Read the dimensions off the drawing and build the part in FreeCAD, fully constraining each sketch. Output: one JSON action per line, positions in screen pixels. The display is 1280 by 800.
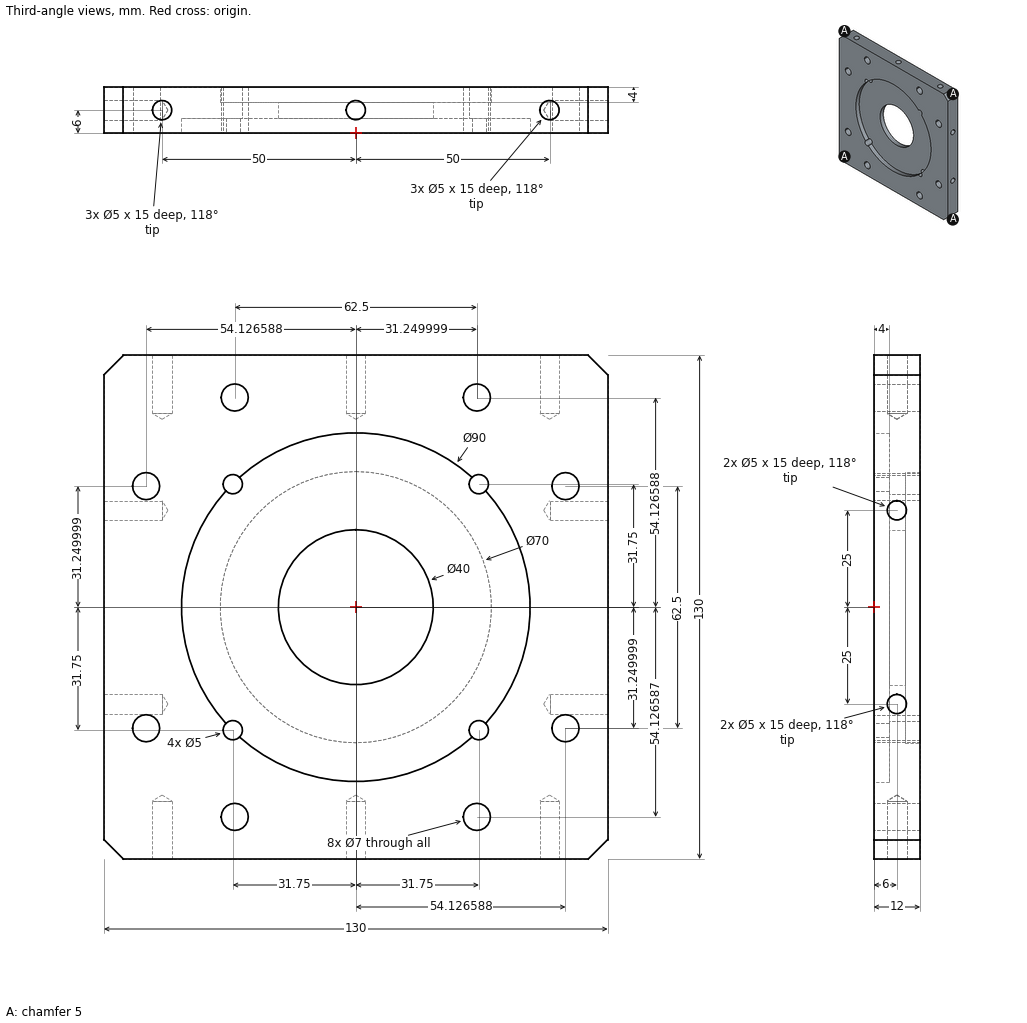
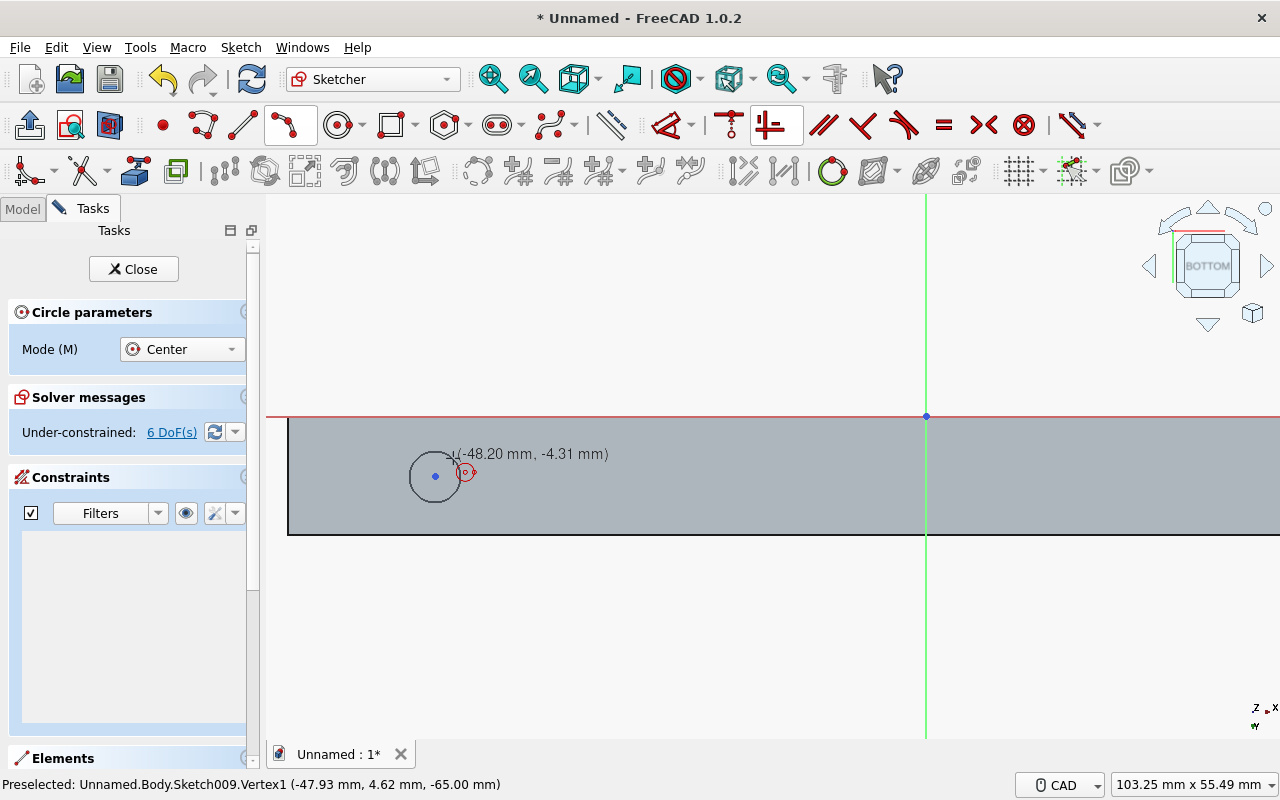
{"action": "left_click", "coordinate": [926, 476]}
{"action": "left_click", "coordinate": [944, 458]}
{"action": "key", "text": "Escape"}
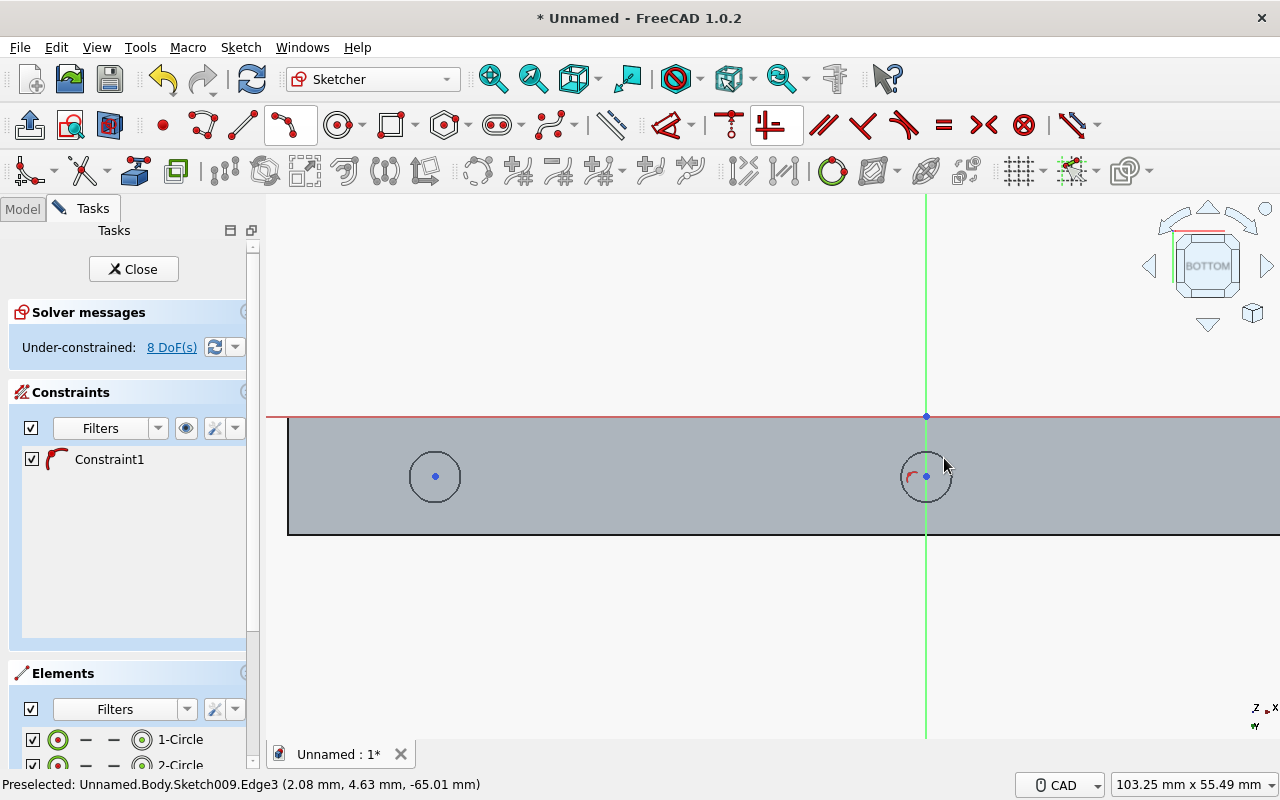
{"action": "scroll", "coordinate": [435, 476], "scroll_direction": "down", "scroll_amount": 3}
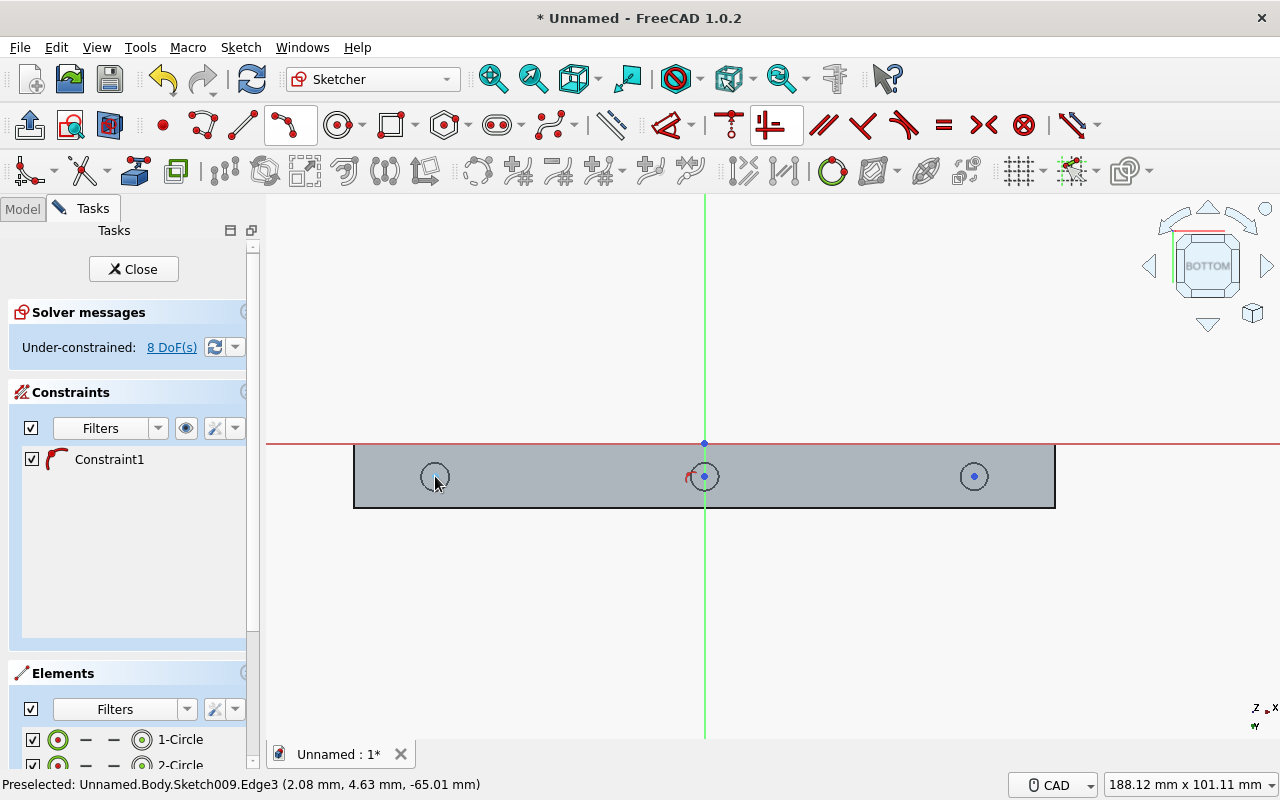
{"action": "left_click", "coordinate": [984, 467]}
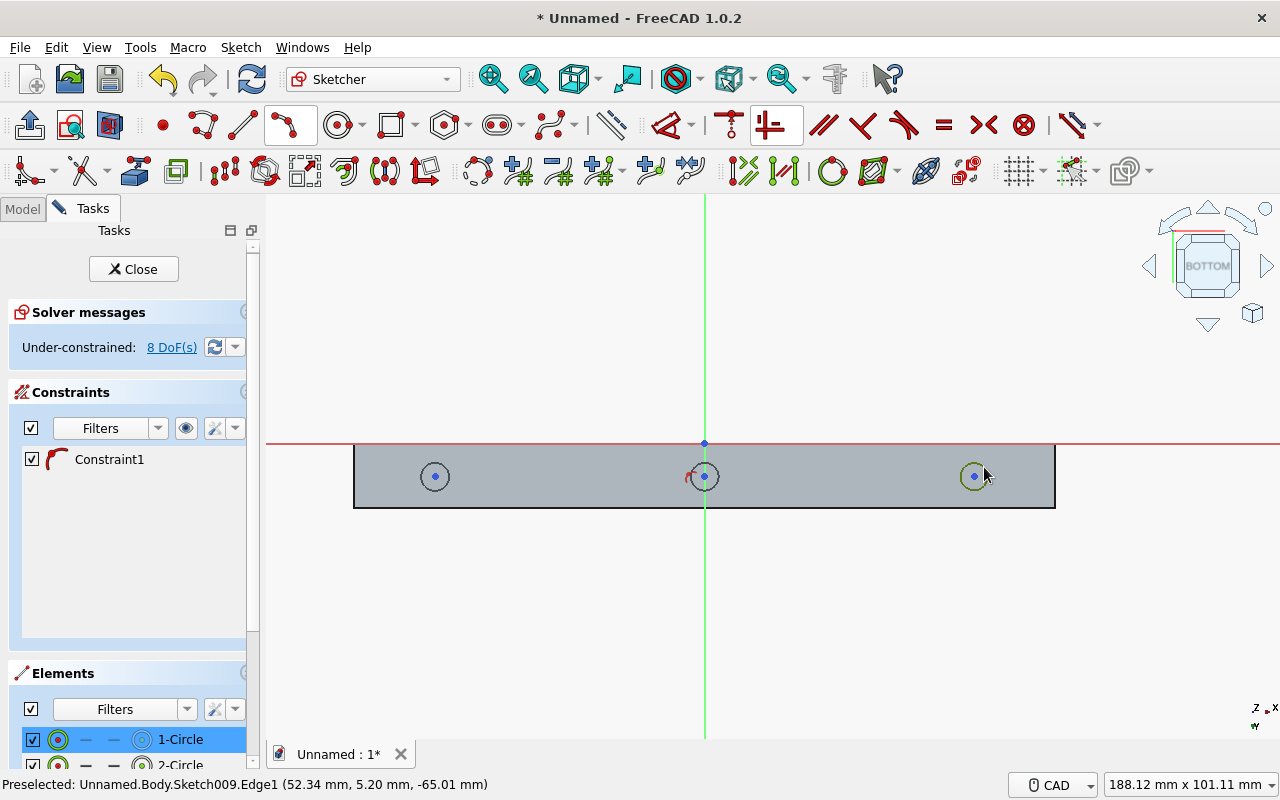
{"action": "left_click", "coordinate": [445, 467]}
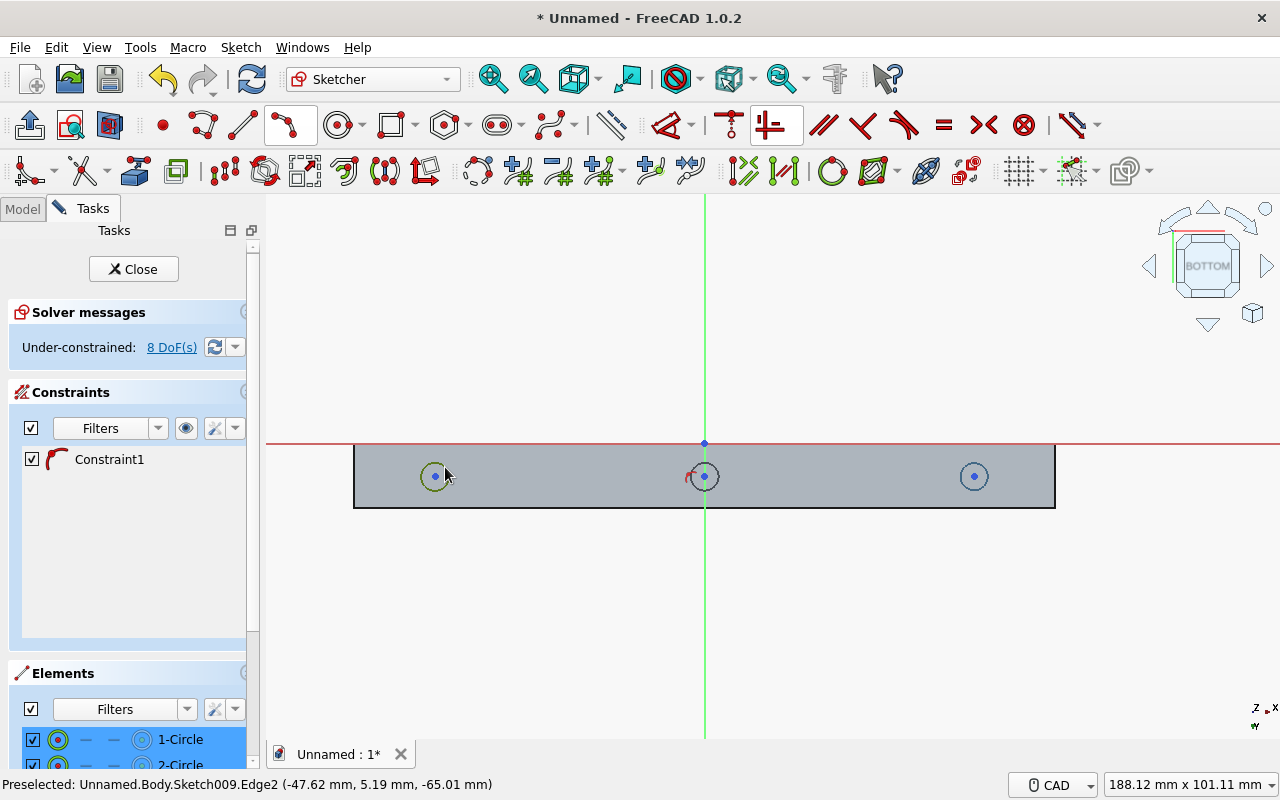
{"action": "scroll", "coordinate": [714, 467], "scroll_direction": "up", "scroll_amount": 2}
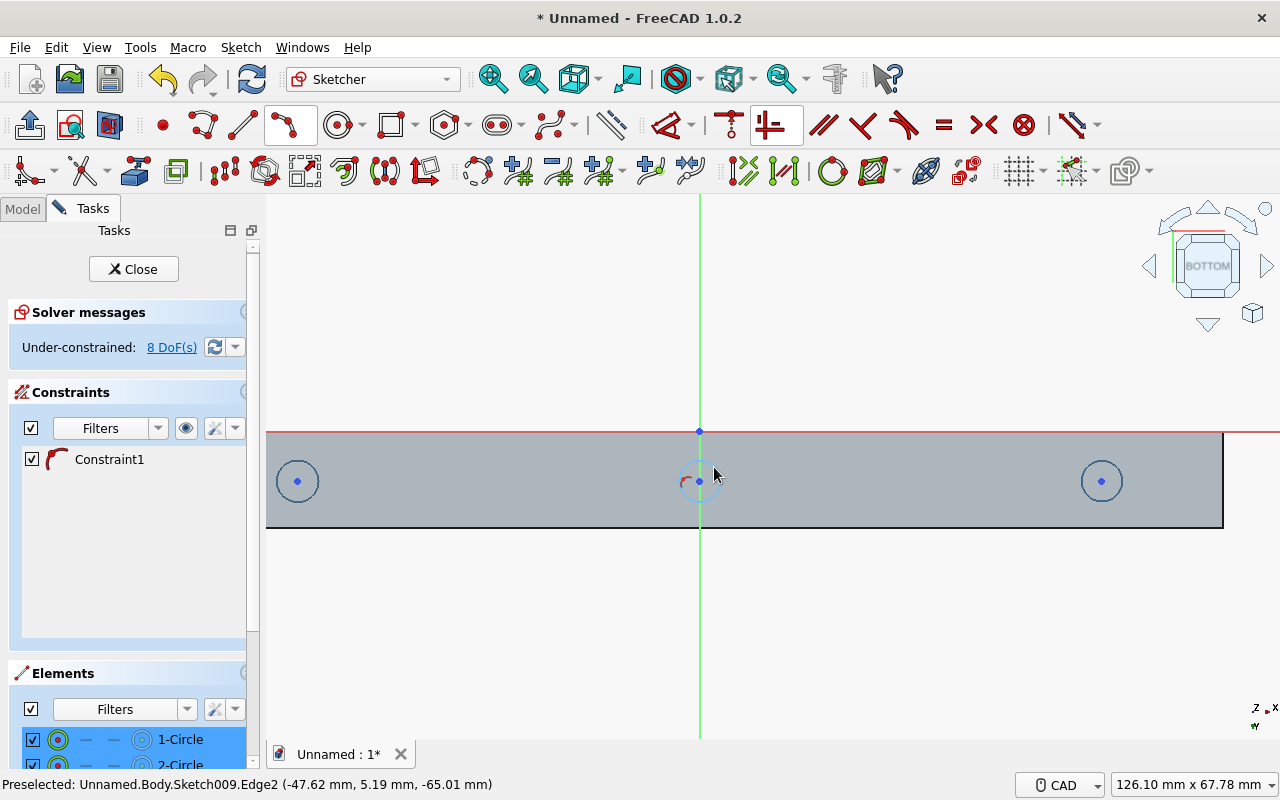
{"action": "left_click", "coordinate": [715, 467]}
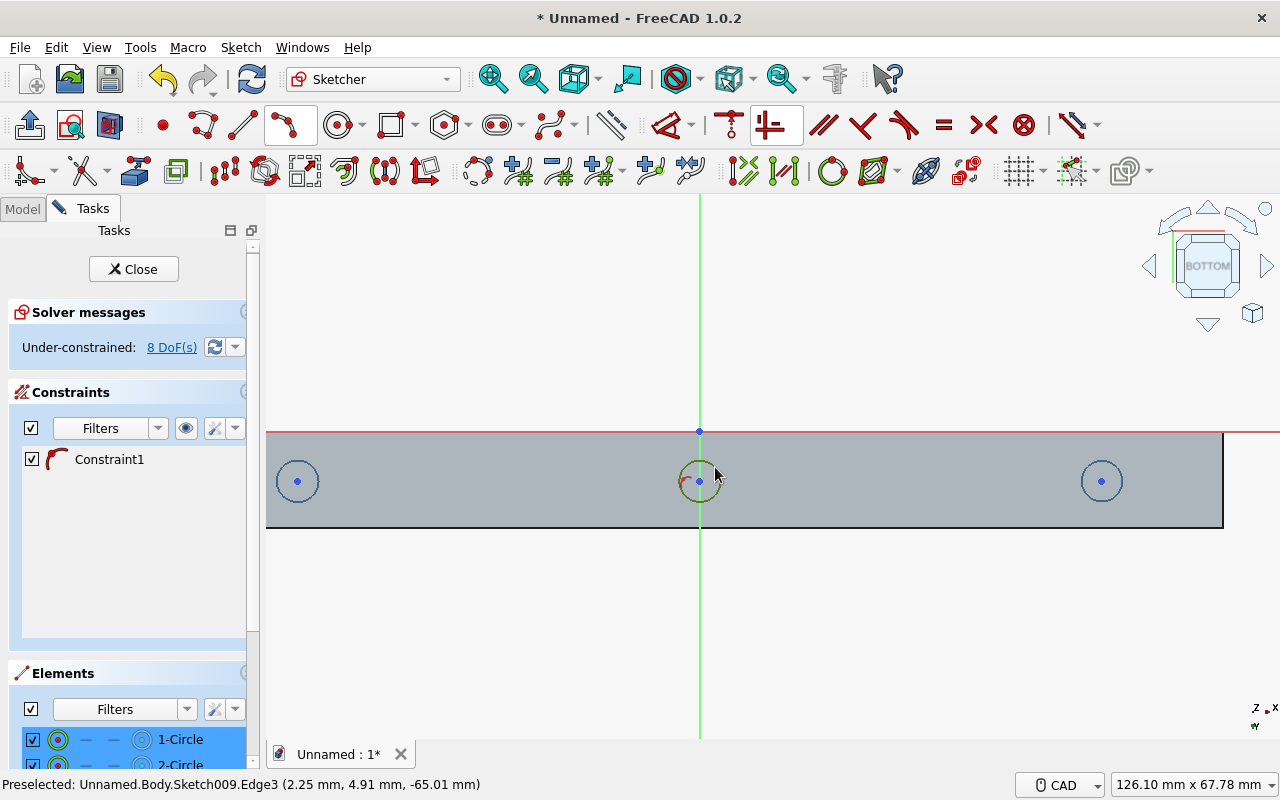
{"action": "key", "text": "e"}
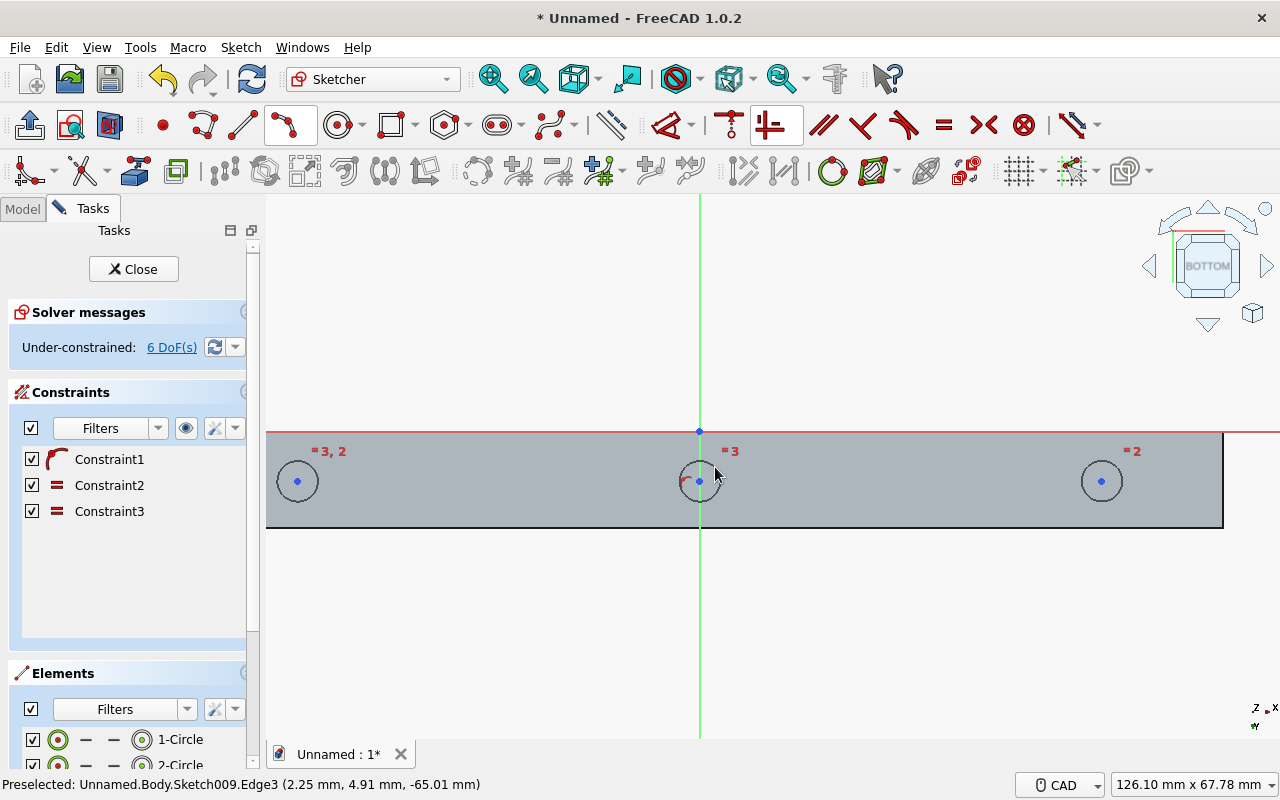
{"action": "left_click", "coordinate": [1102, 481]}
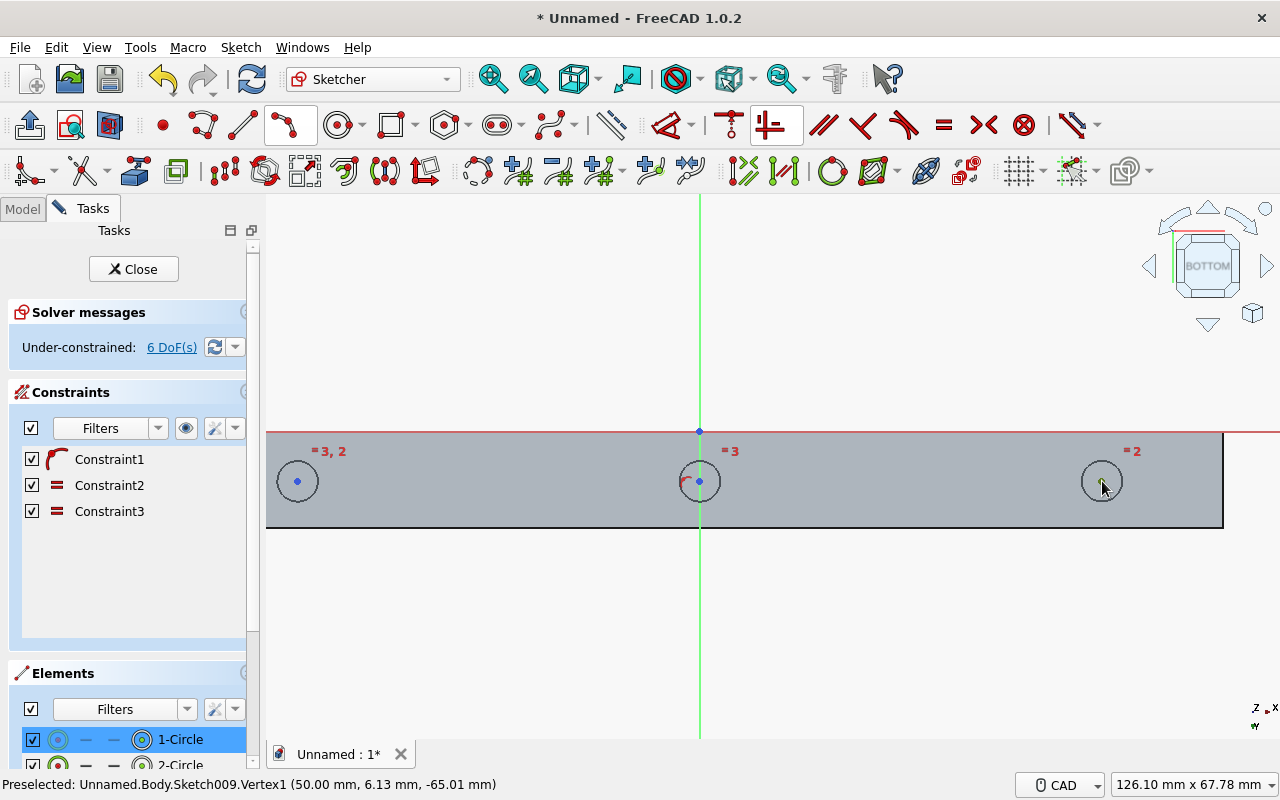
{"action": "left_click", "coordinate": [298, 481]}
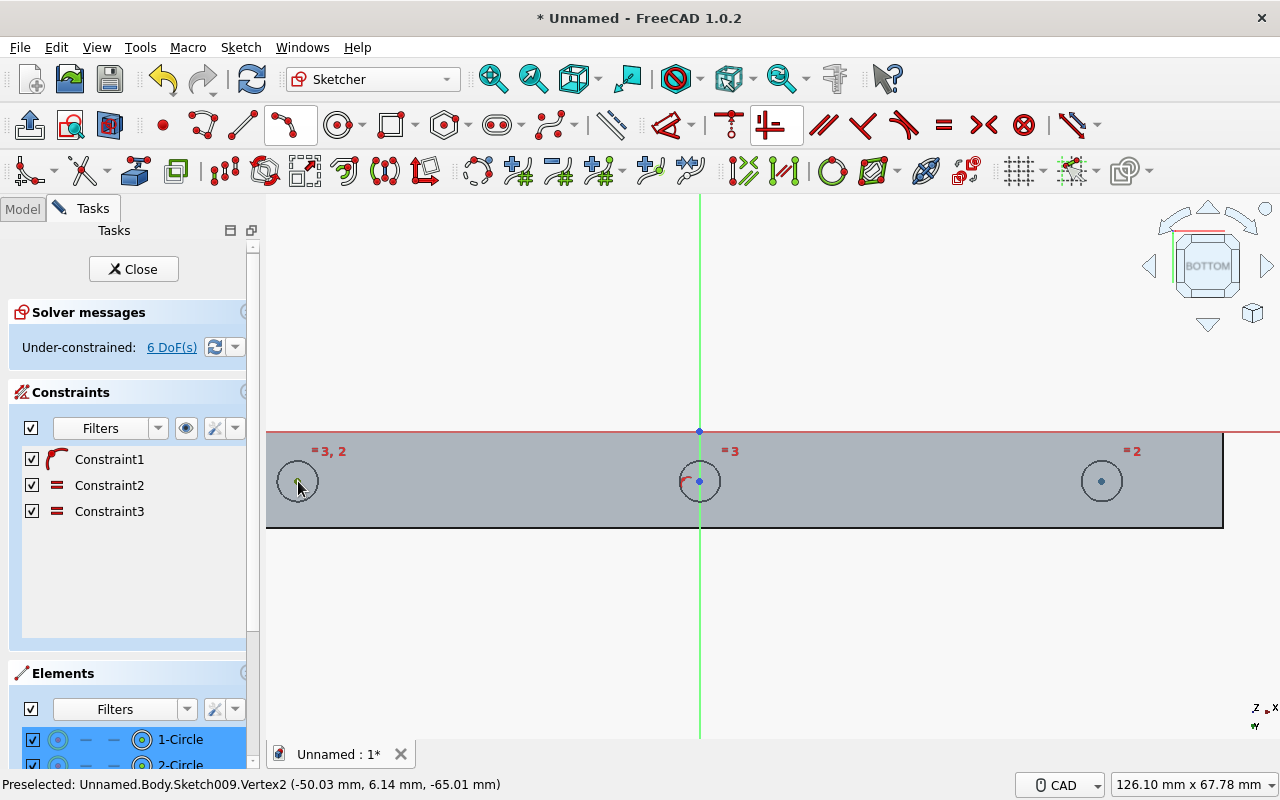
{"action": "key", "text": "h"}